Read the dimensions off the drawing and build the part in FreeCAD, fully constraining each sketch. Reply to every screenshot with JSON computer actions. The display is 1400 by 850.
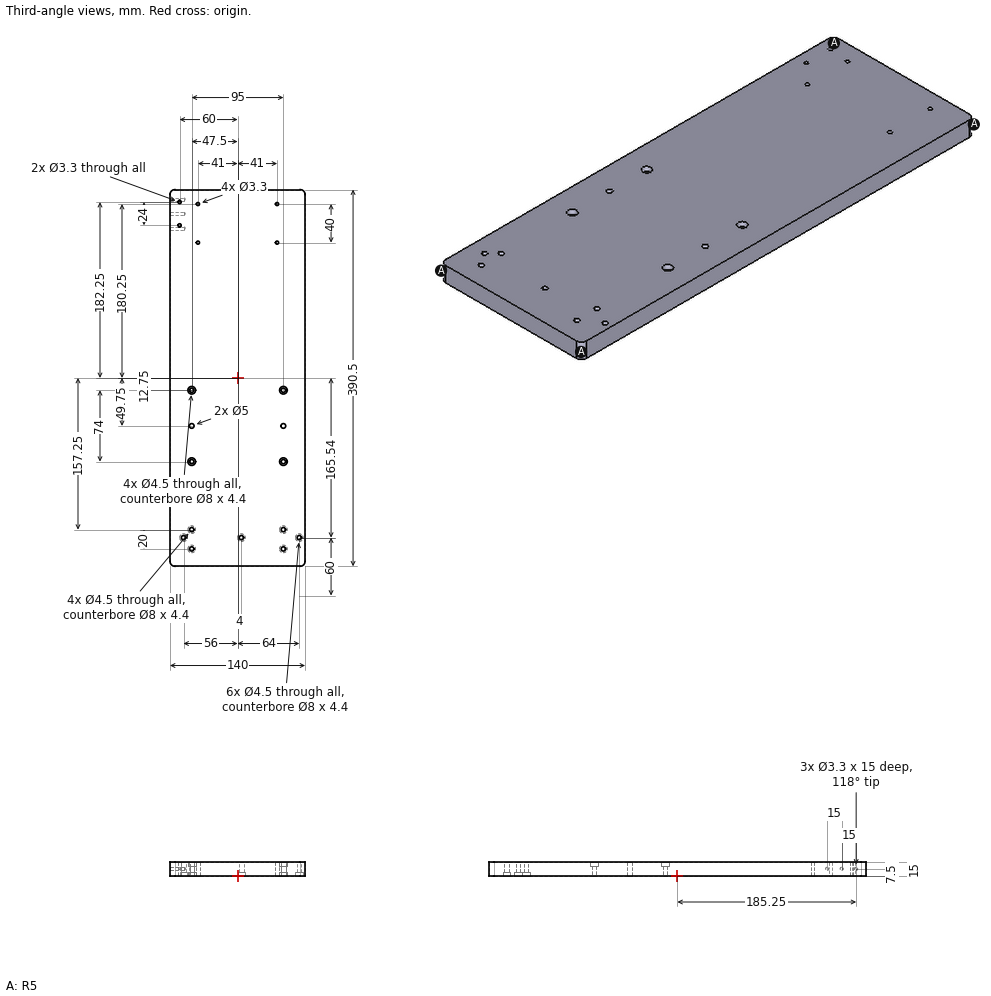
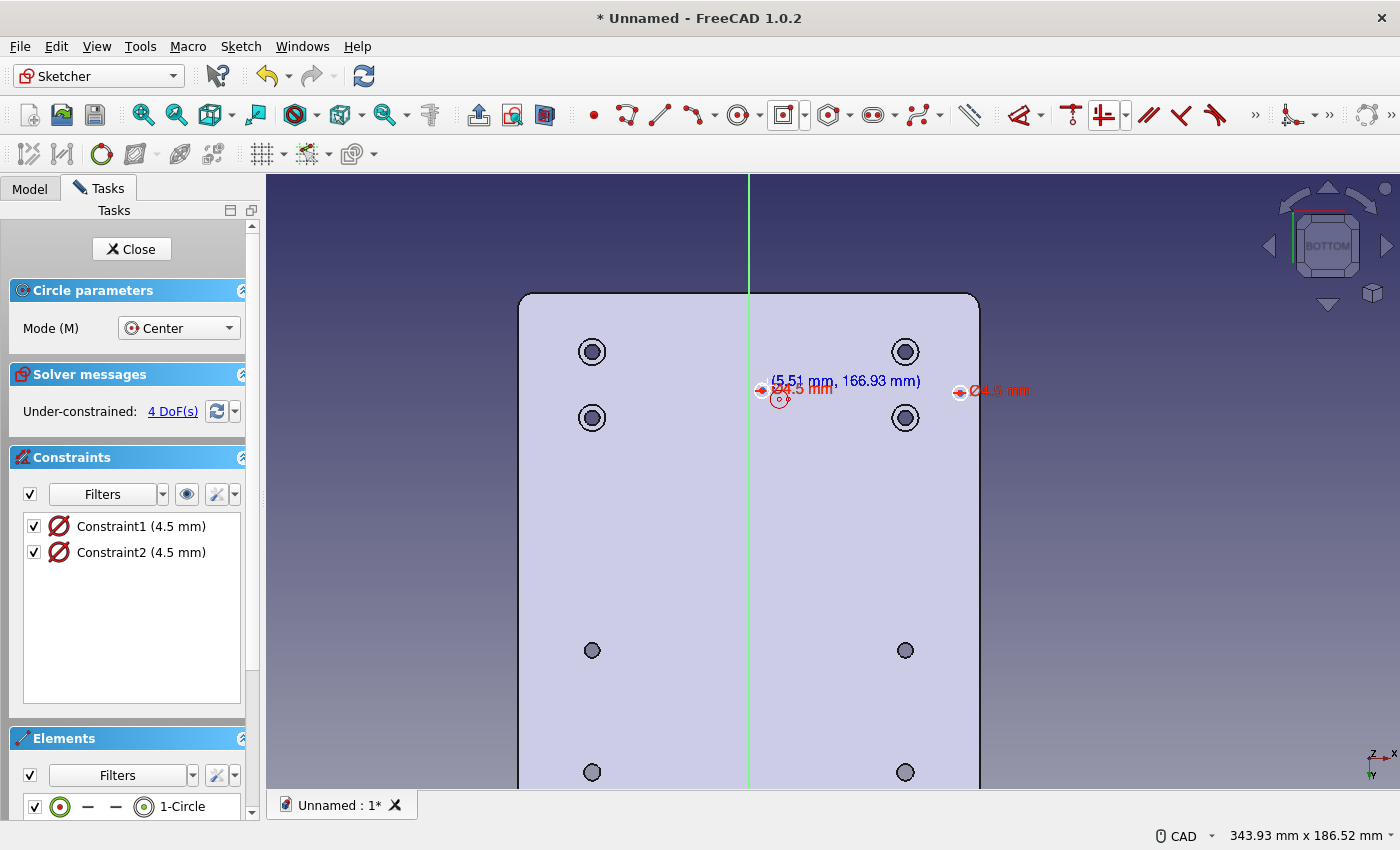
{"action": "scroll", "coordinate": [767, 385], "scroll_direction": "down", "scroll_amount": 3}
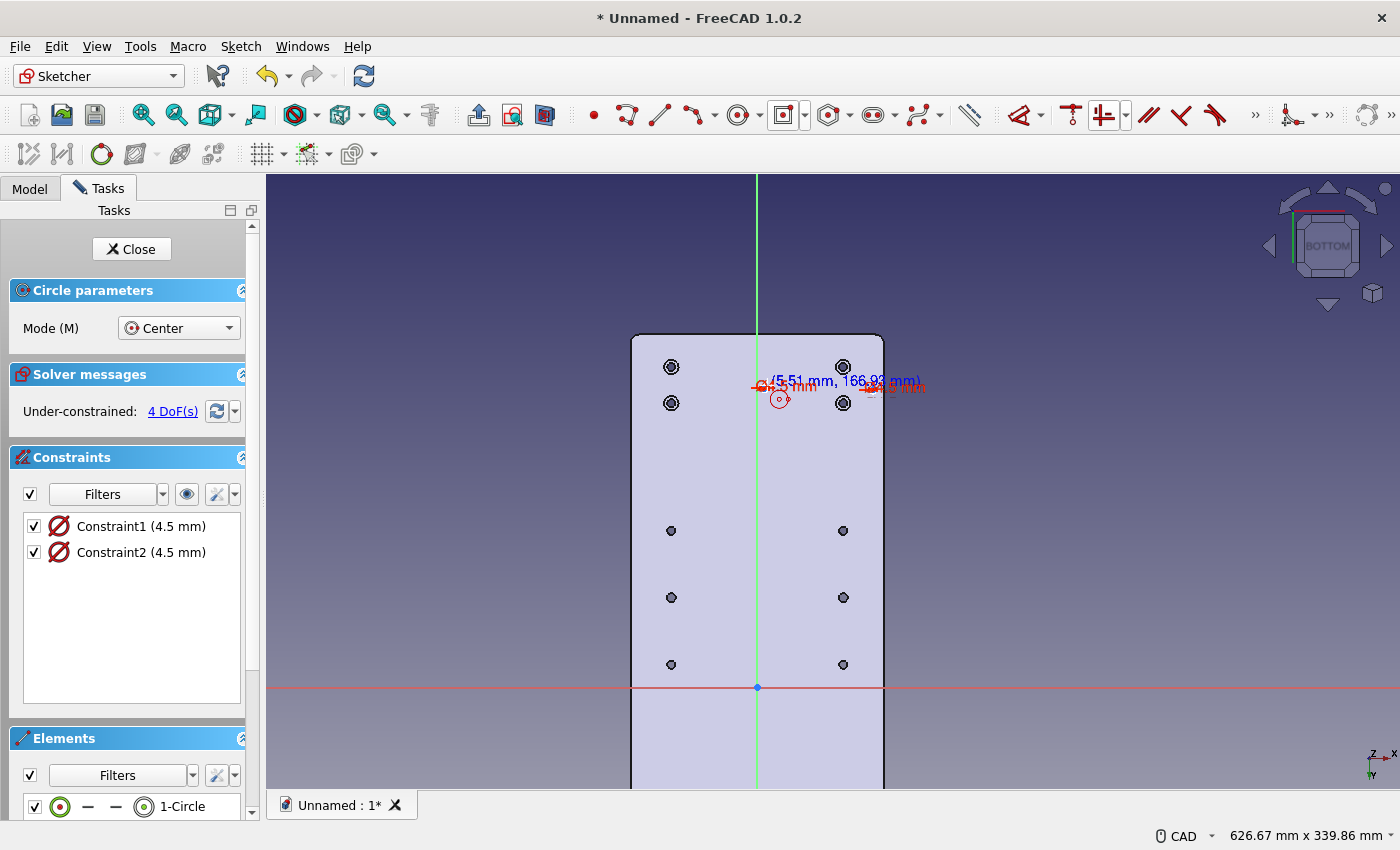
{"action": "scroll", "coordinate": [873, 280], "scroll_direction": "up", "scroll_amount": 9}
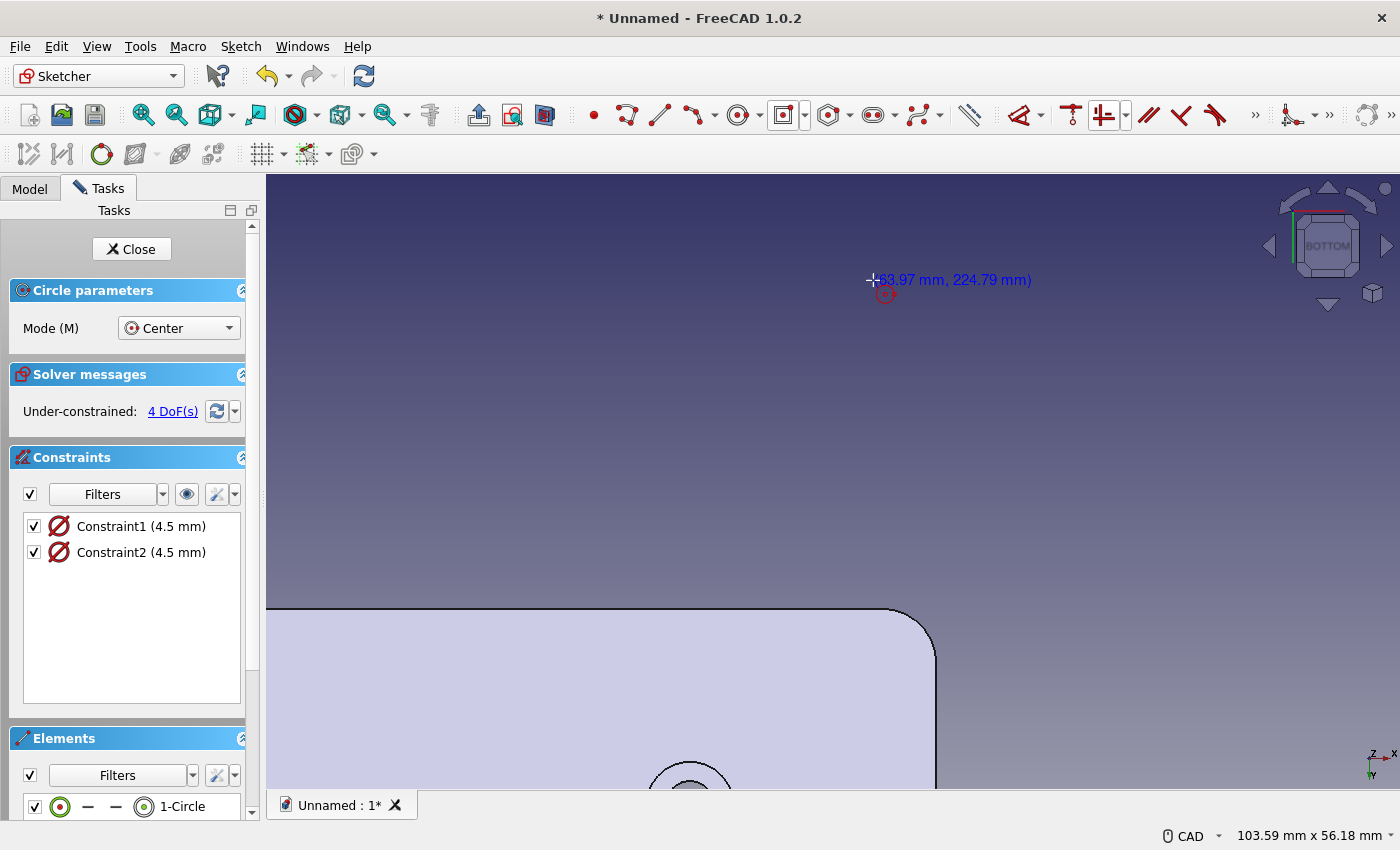
{"action": "scroll", "coordinate": [874, 280], "scroll_direction": "down", "scroll_amount": 9}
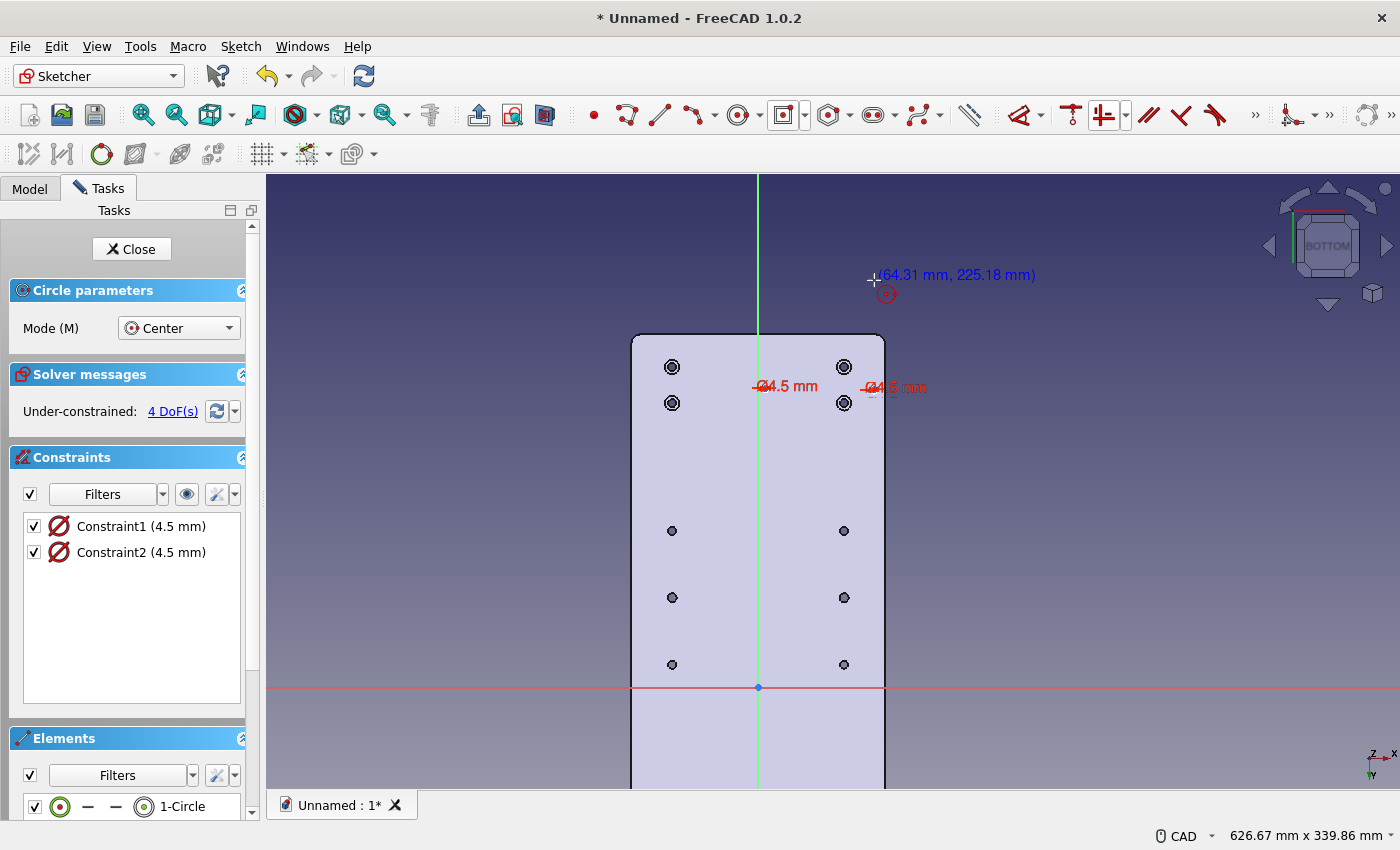
{"action": "left_click", "coordinate": [874, 280]}
{"action": "mouse_move", "coordinate": [877, 277]}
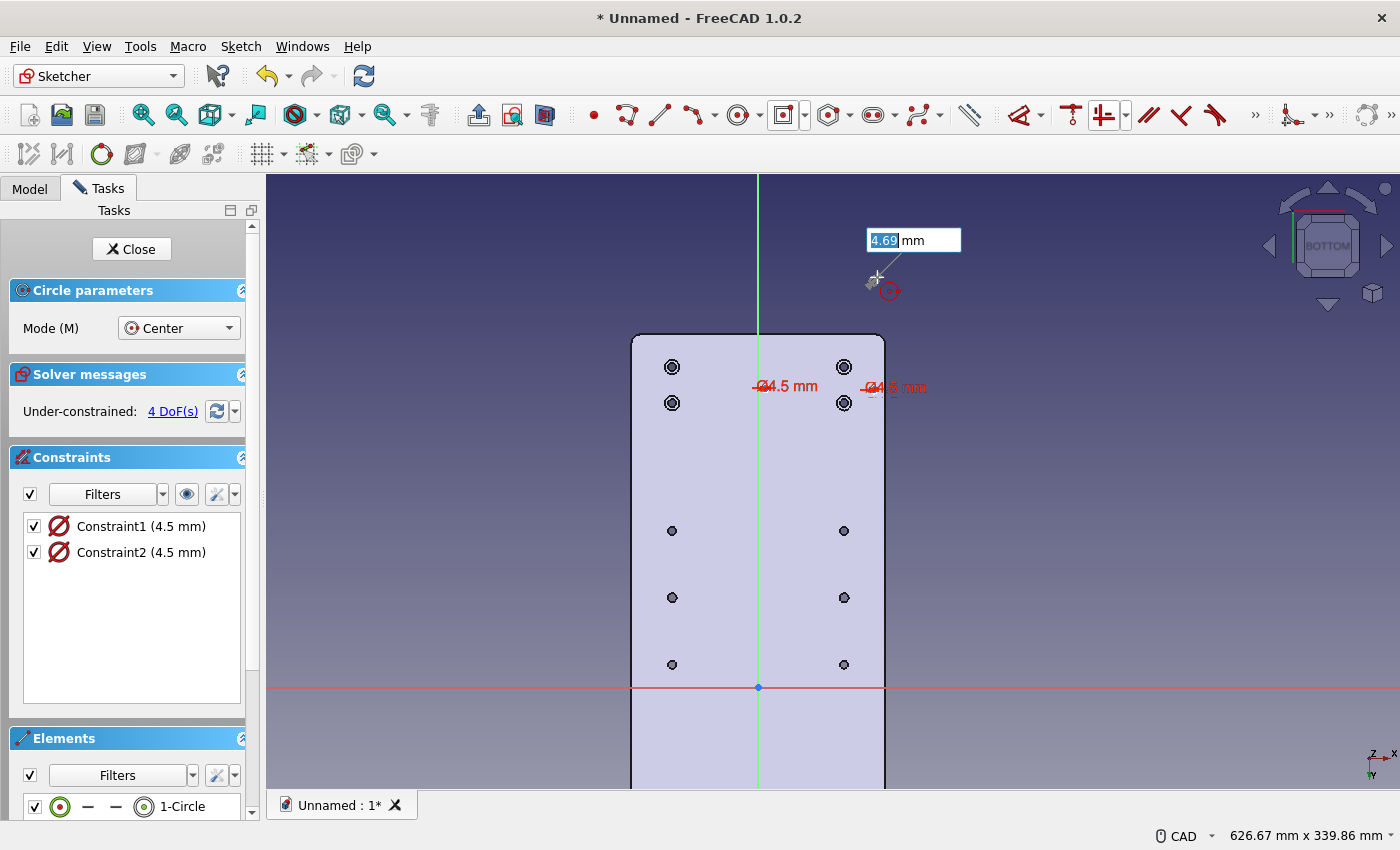
{"action": "type", "text": "4.5"}
{"action": "key", "text": "Return"}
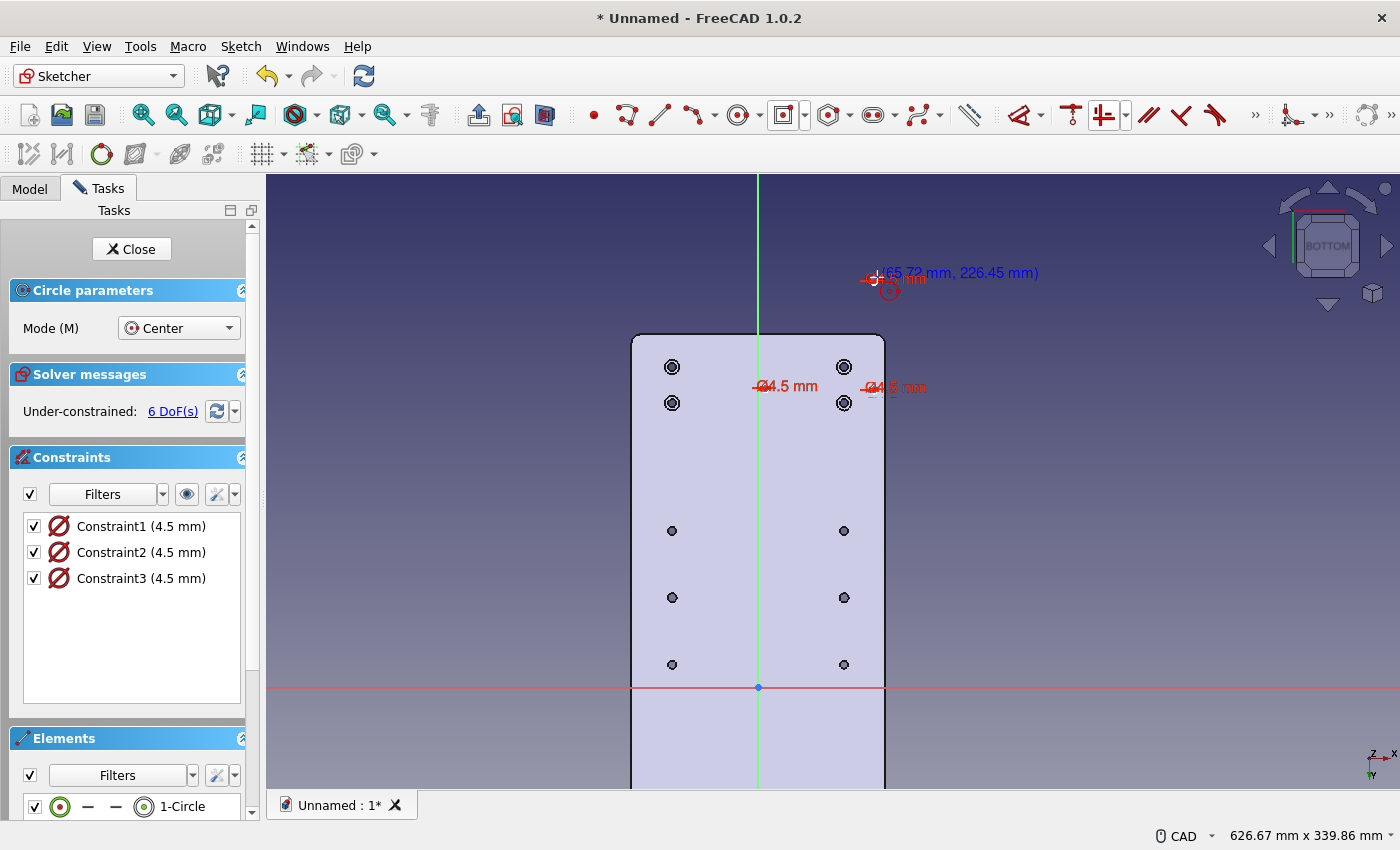
{"action": "scroll", "coordinate": [765, 280], "scroll_direction": "up", "scroll_amount": 9}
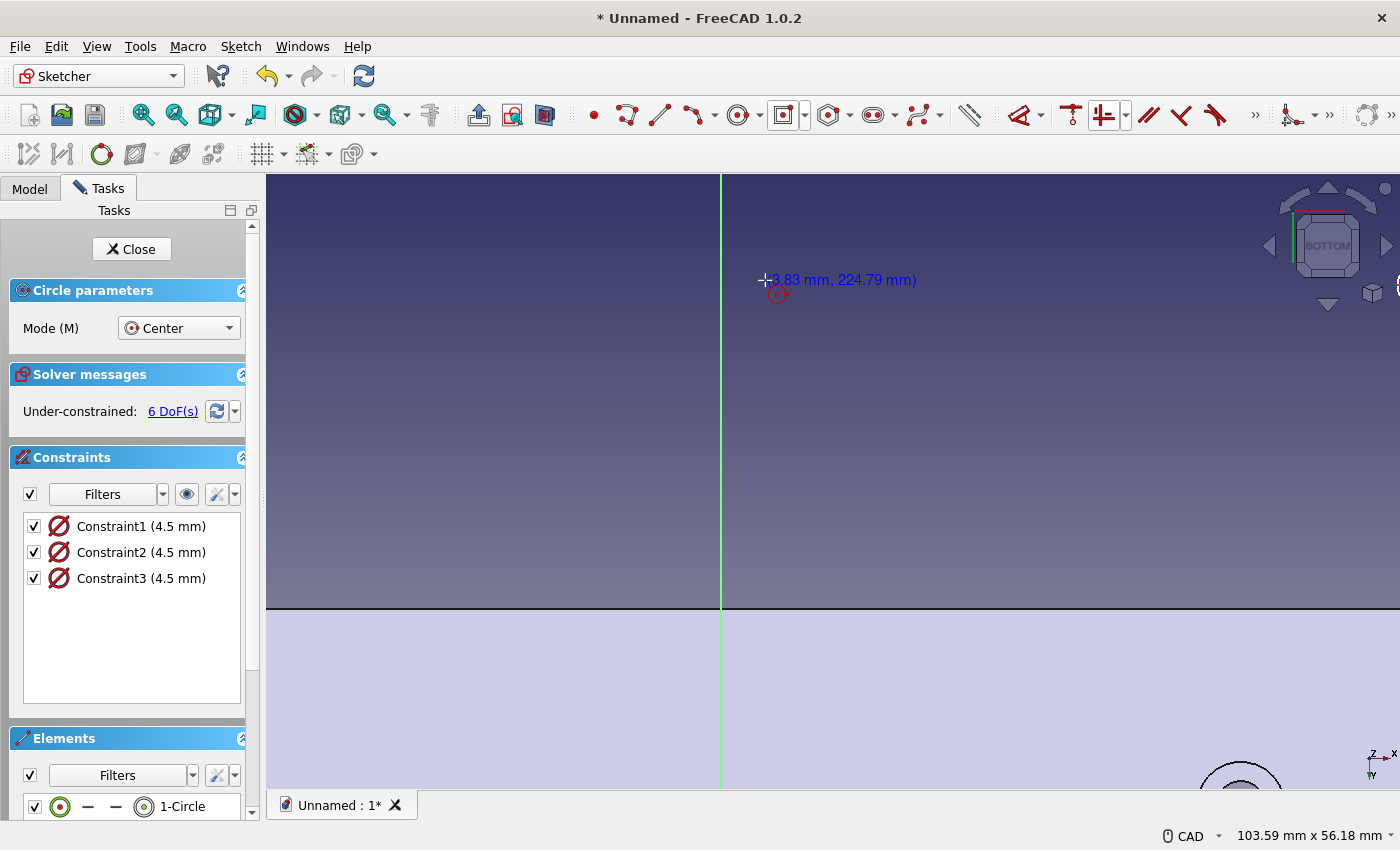
{"action": "left_click", "coordinate": [765, 277]}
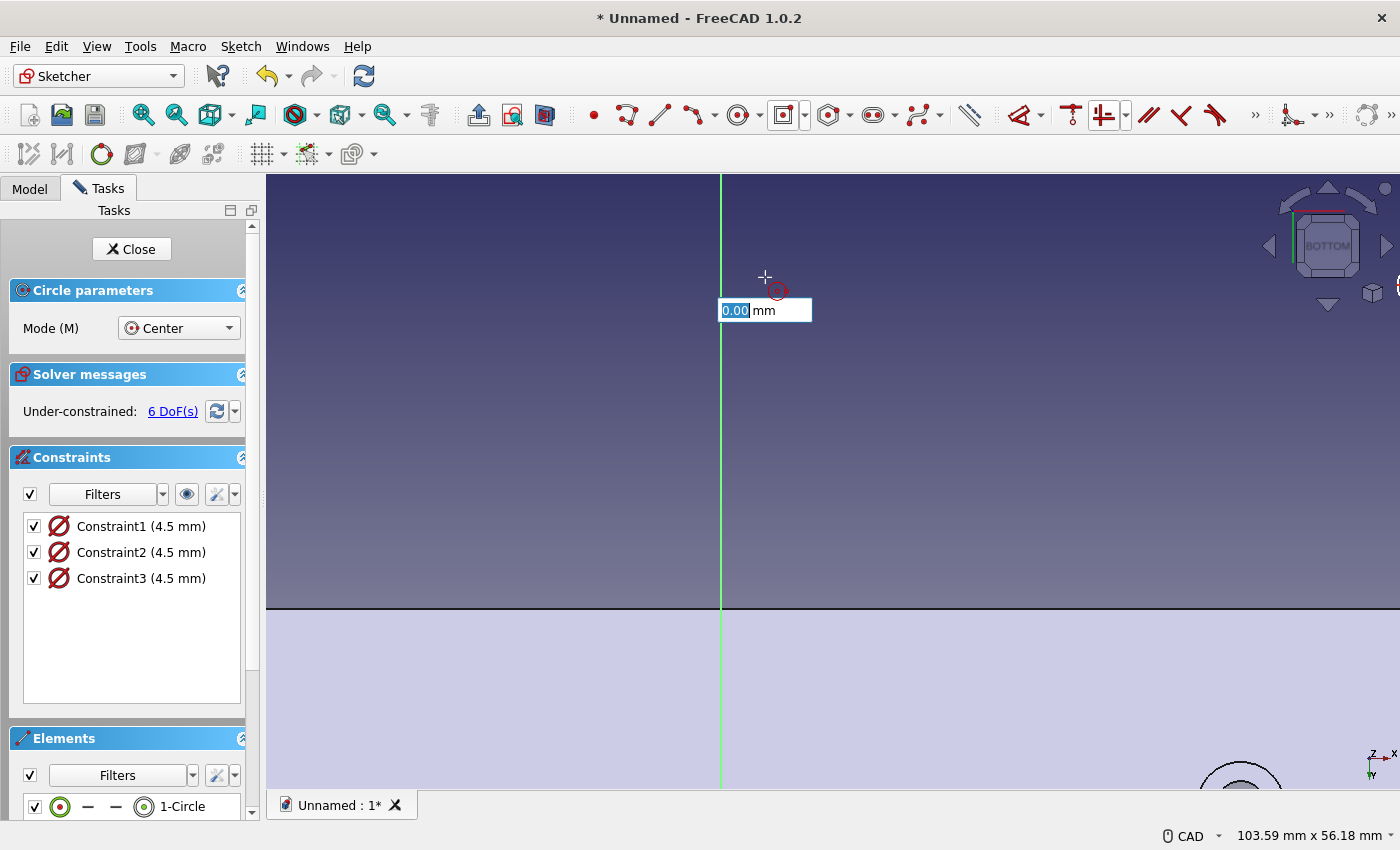
{"action": "scroll", "coordinate": [764, 280], "scroll_direction": "down", "scroll_amount": 9}